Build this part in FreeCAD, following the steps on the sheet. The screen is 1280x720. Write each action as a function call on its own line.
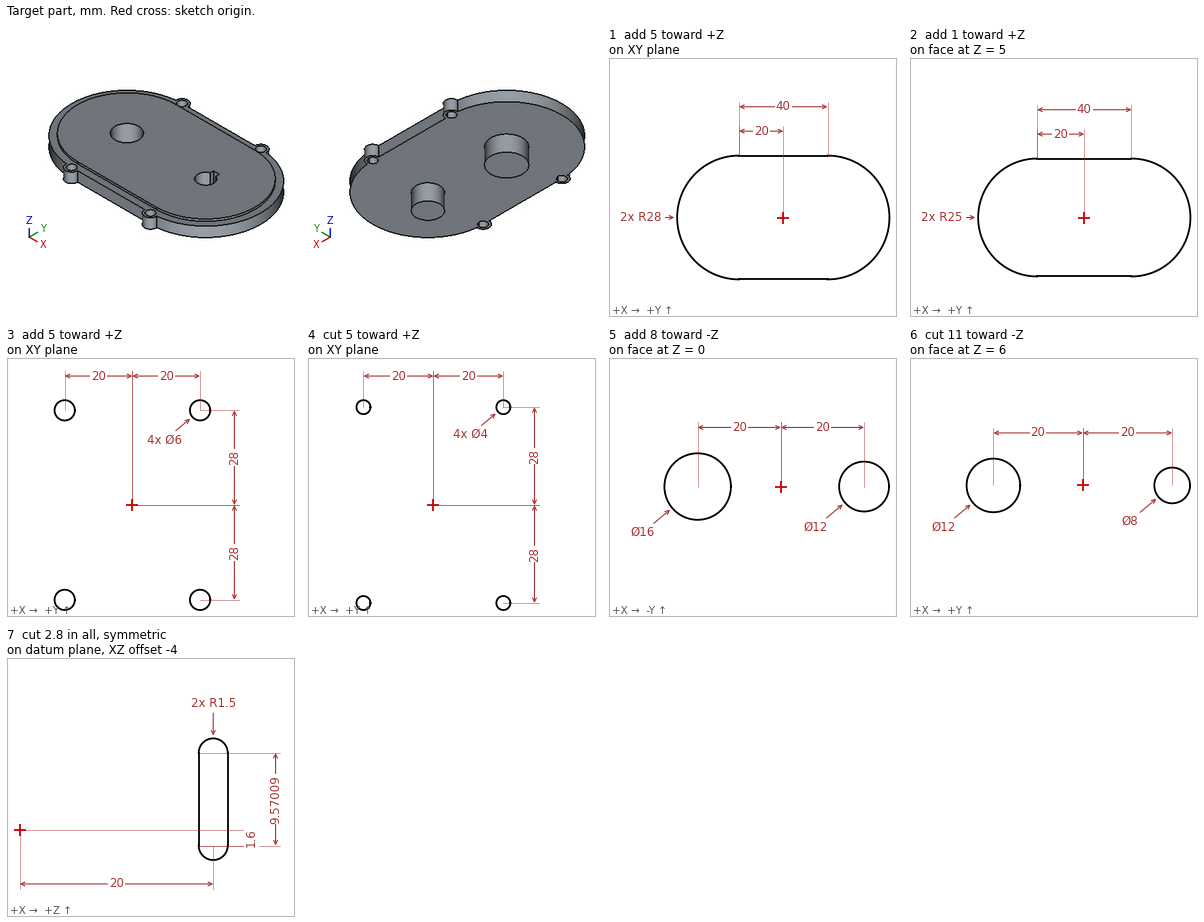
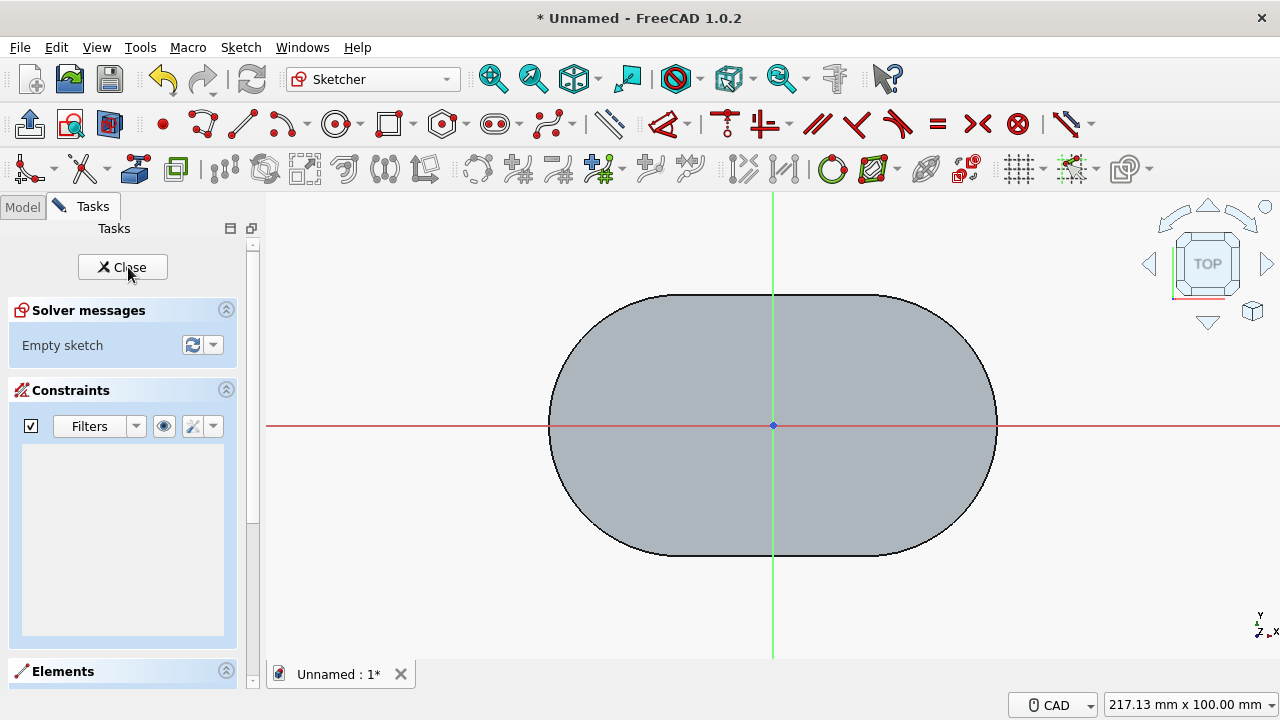
key(g)
key(c)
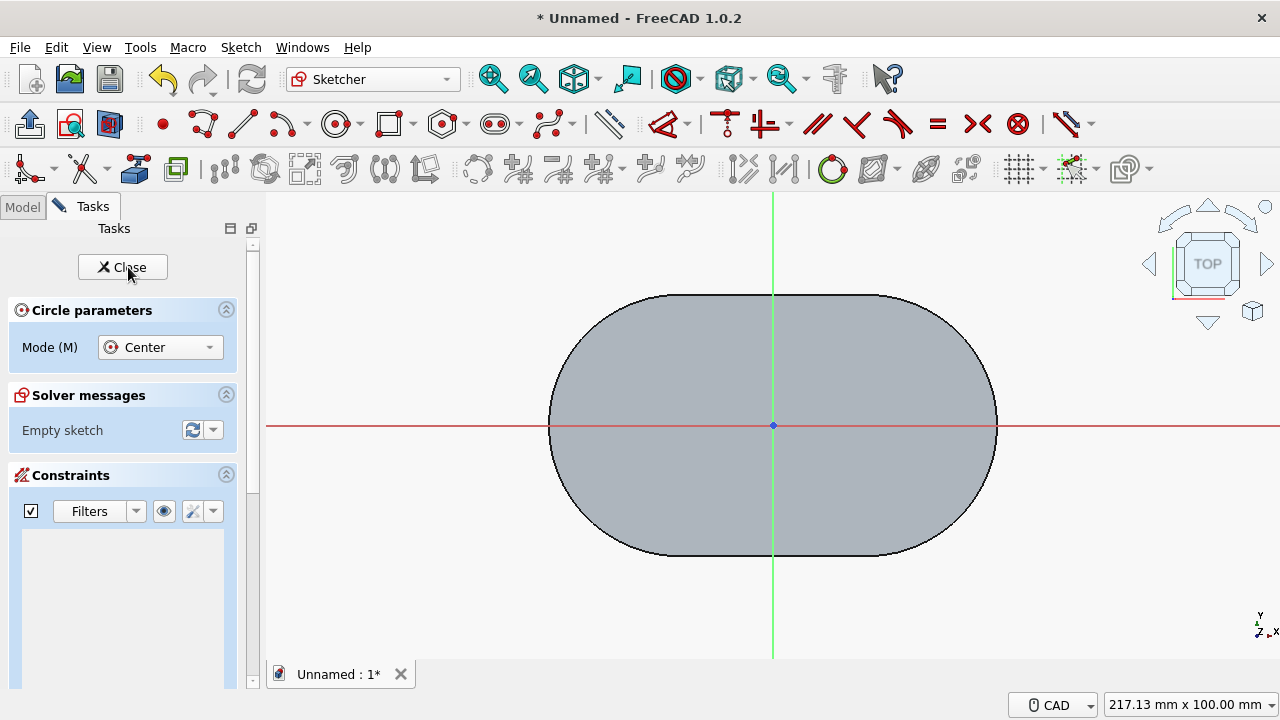
scroll(866, 295, up, 3)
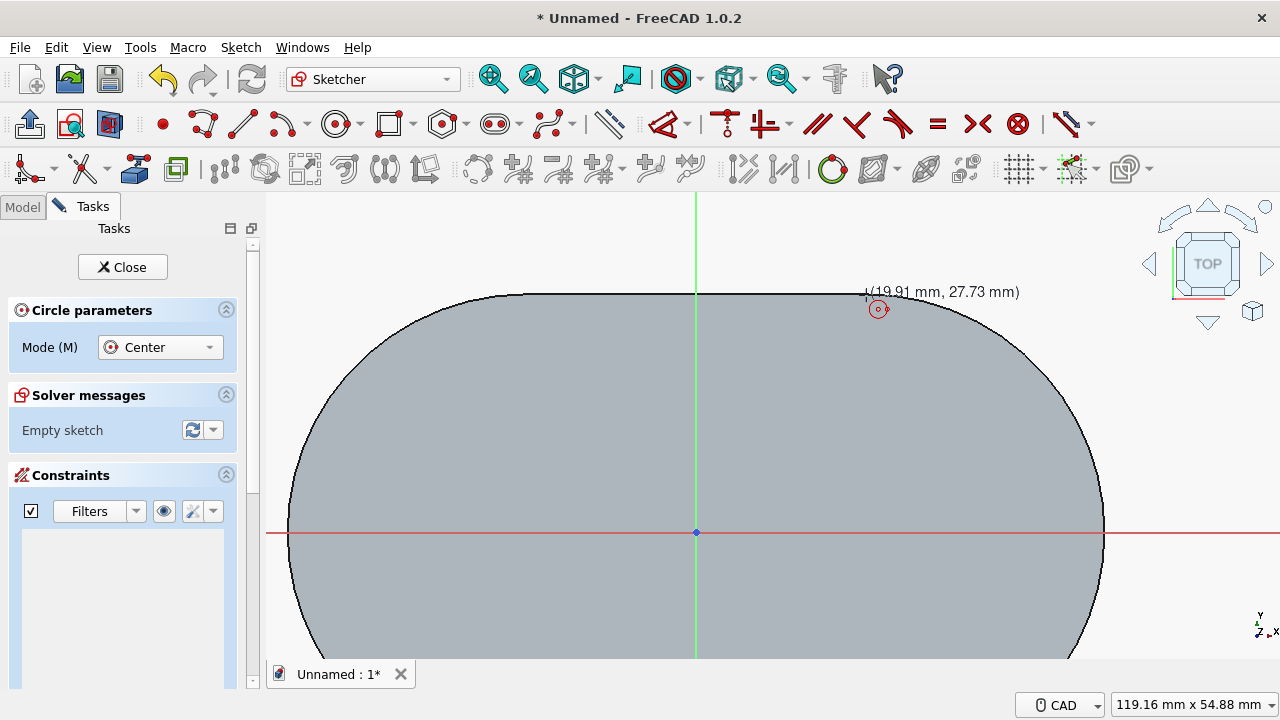
click(866, 294)
click(884, 276)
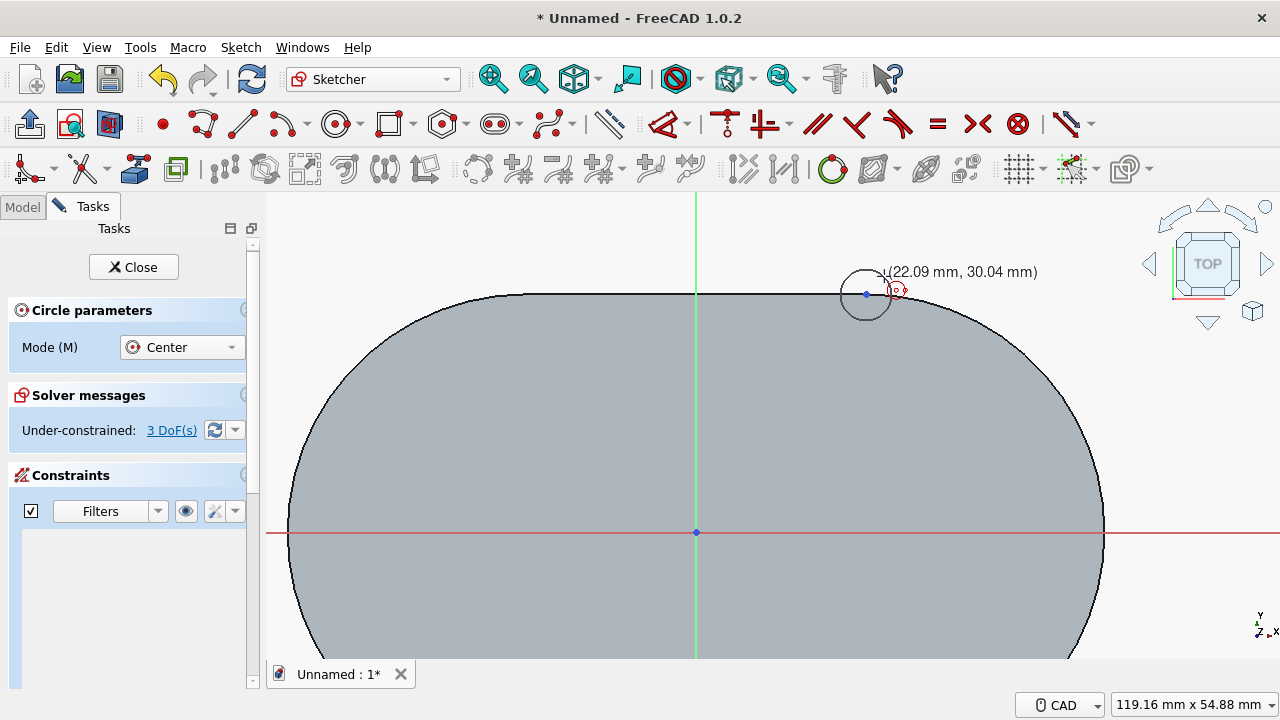
click(526, 294)
click(544, 276)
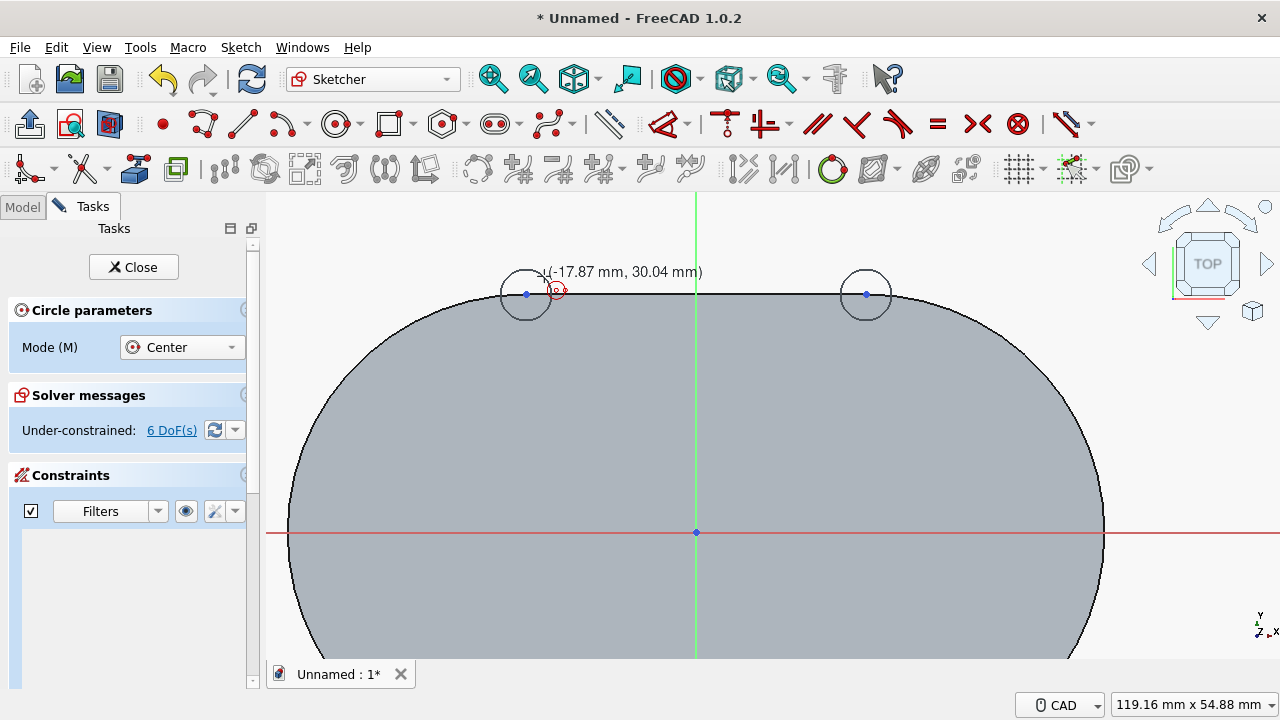
scroll(715, 295, down, 3)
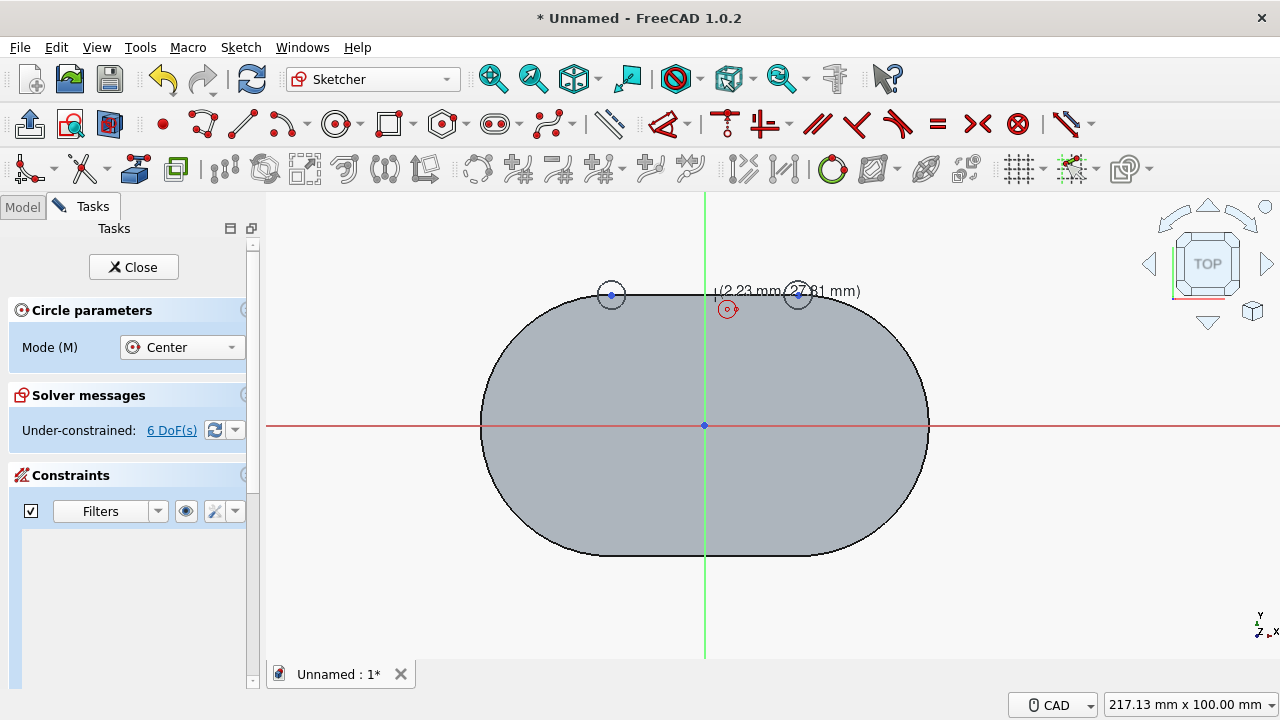
scroll(798, 556, up, 3)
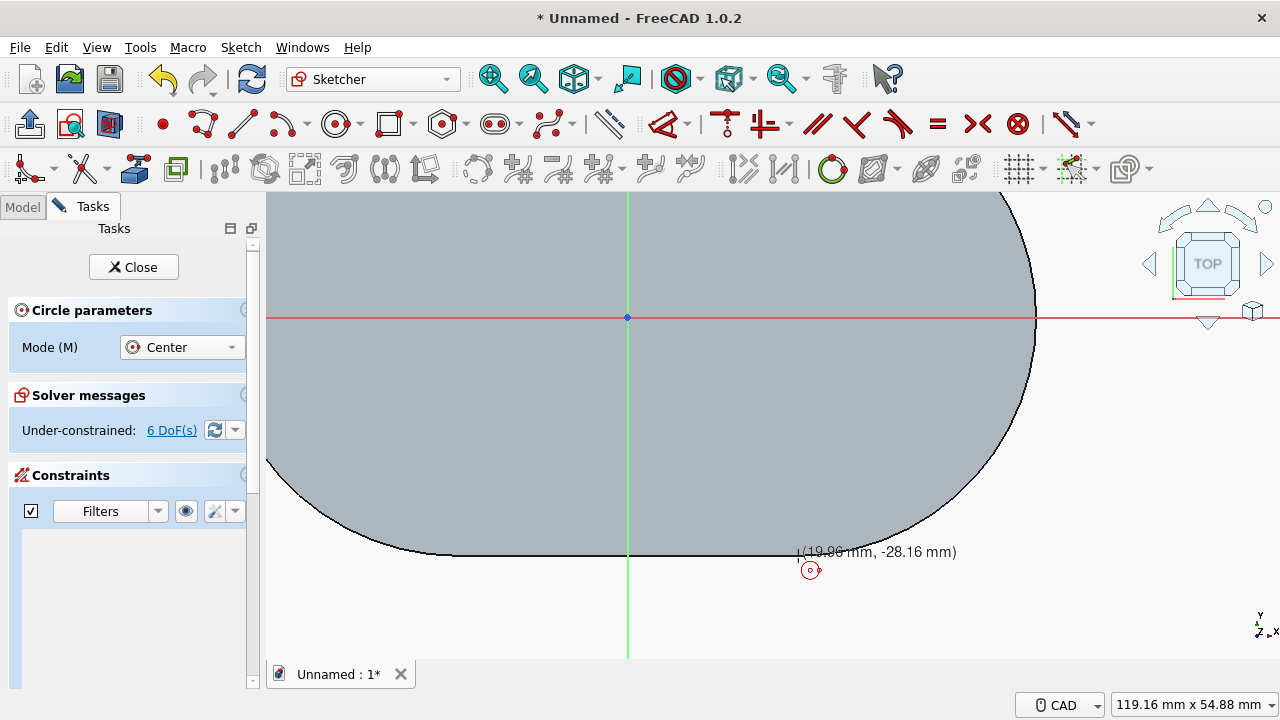
click(798, 556)
click(816, 538)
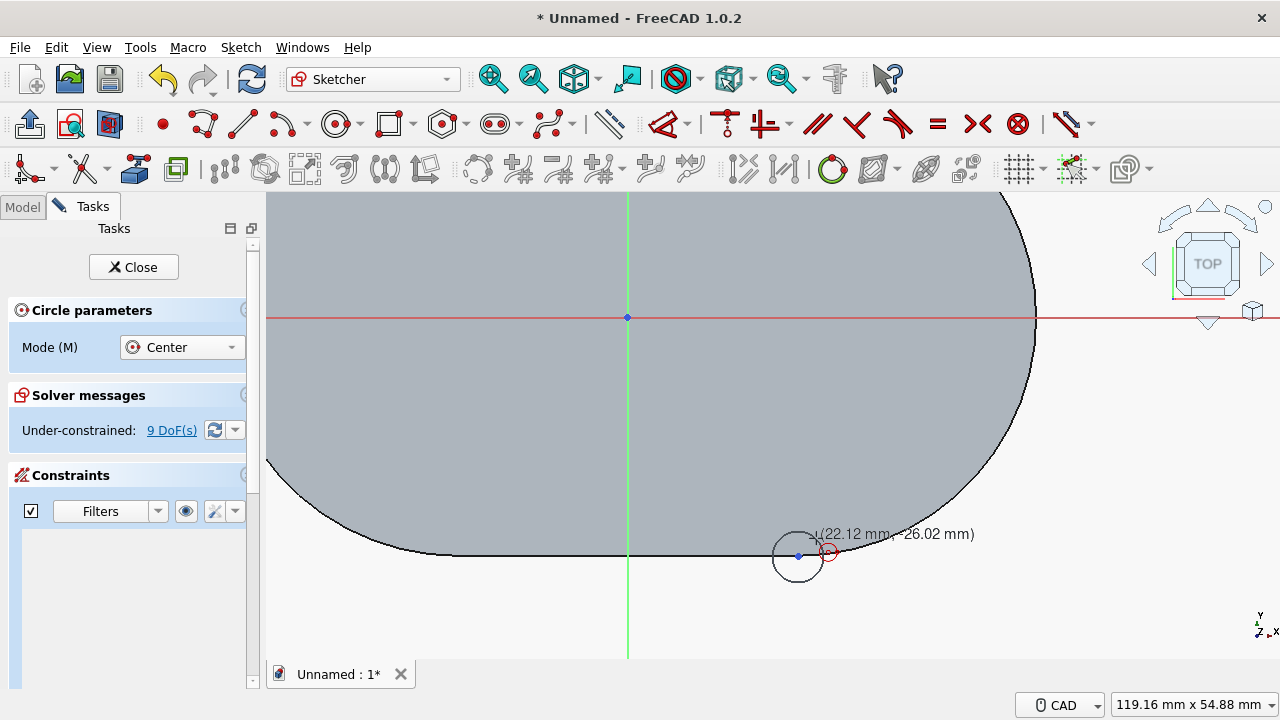
click(458, 556)
click(476, 538)
key(Escape)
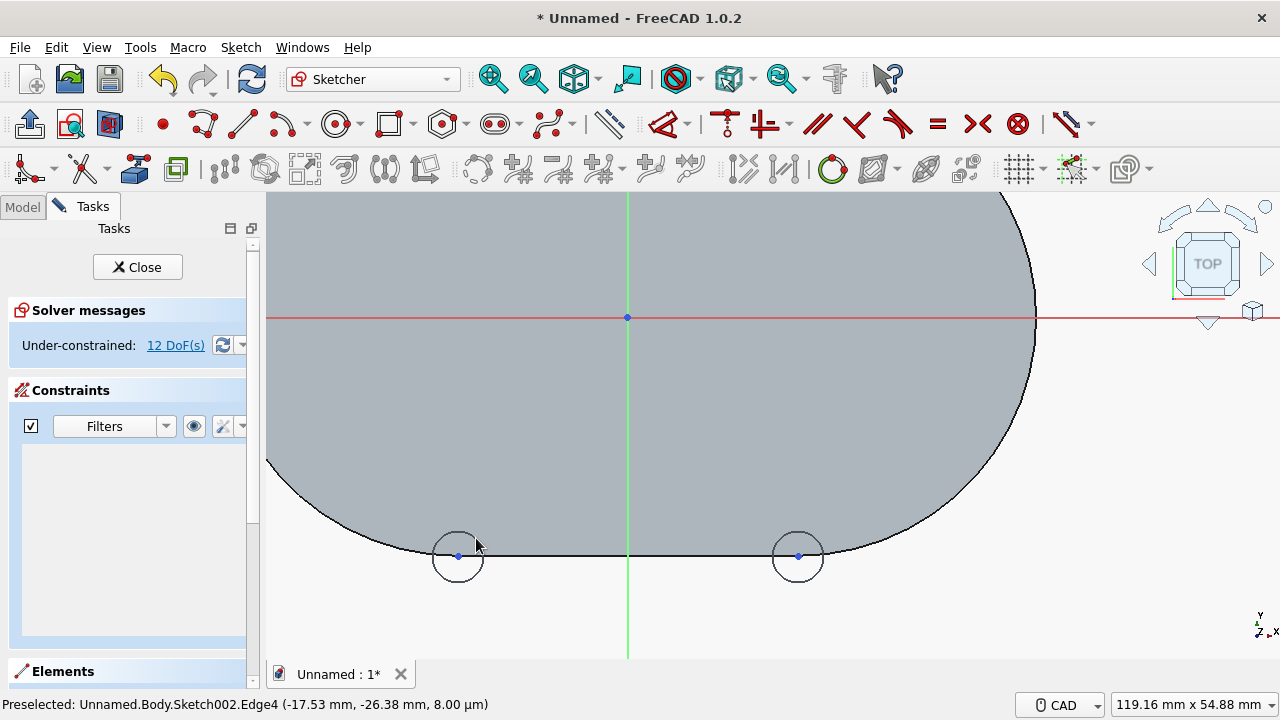
scroll(798, 557, down, 3)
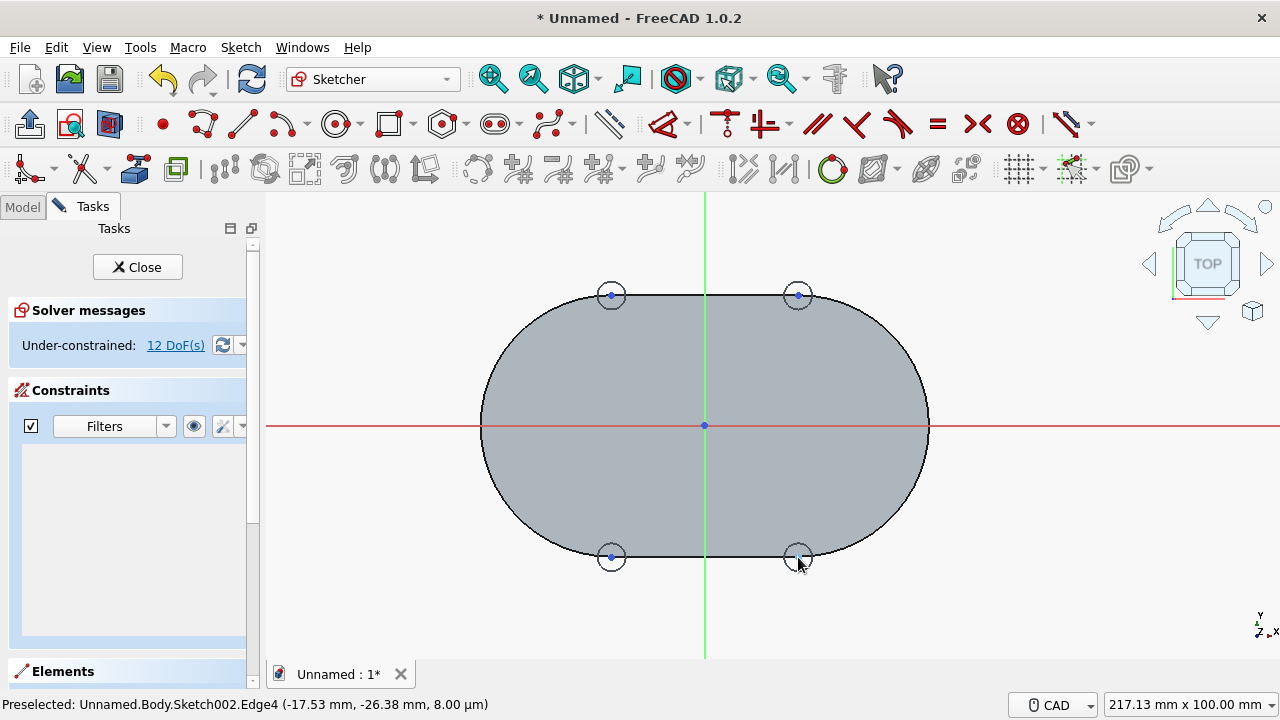
click(808, 286)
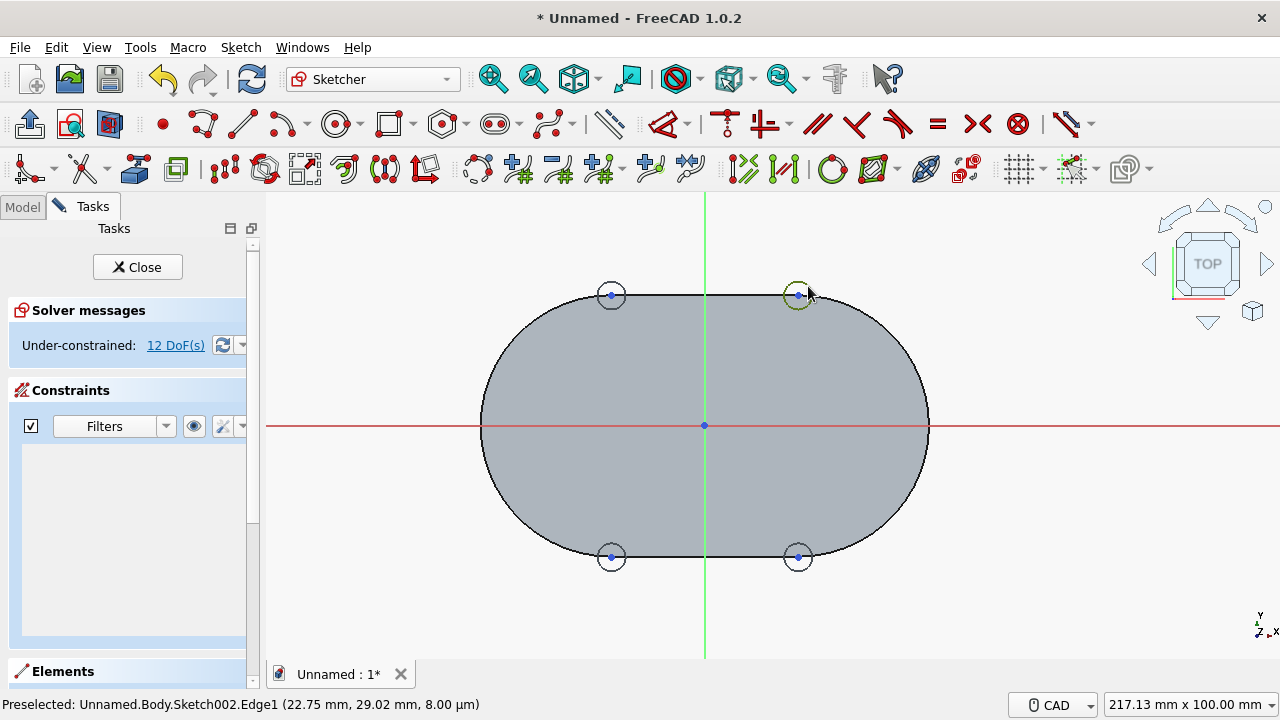
click(621, 286)